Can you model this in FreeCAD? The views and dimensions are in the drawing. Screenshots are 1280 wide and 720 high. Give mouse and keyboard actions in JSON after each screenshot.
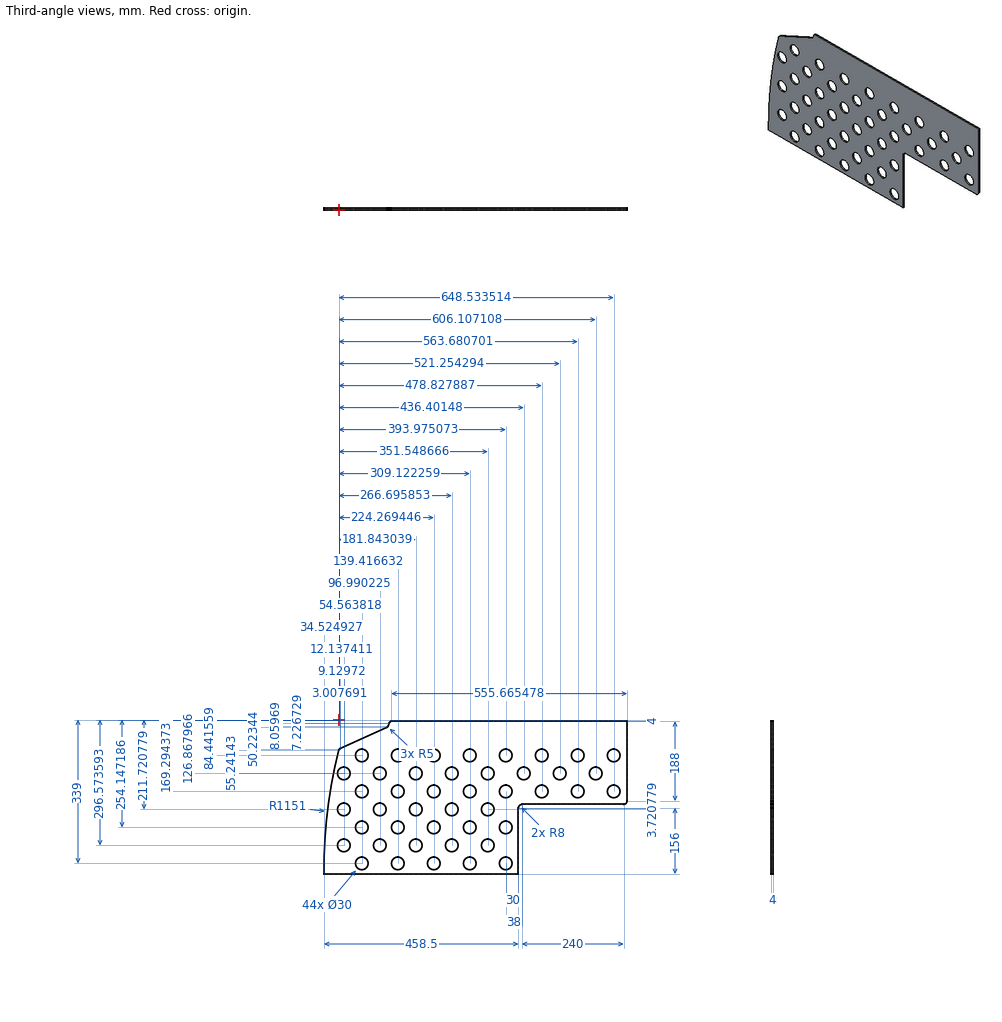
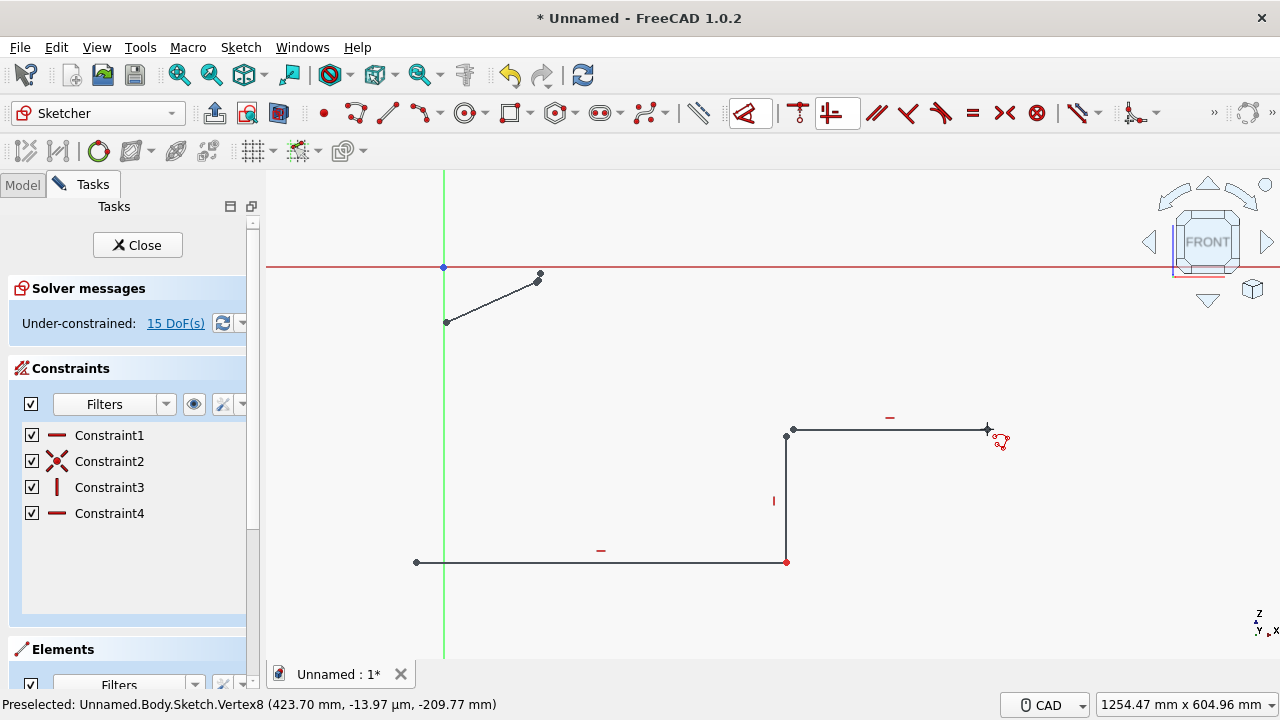
{"action": "scroll", "coordinate": [994, 423], "scroll_direction": "up", "scroll_amount": 3}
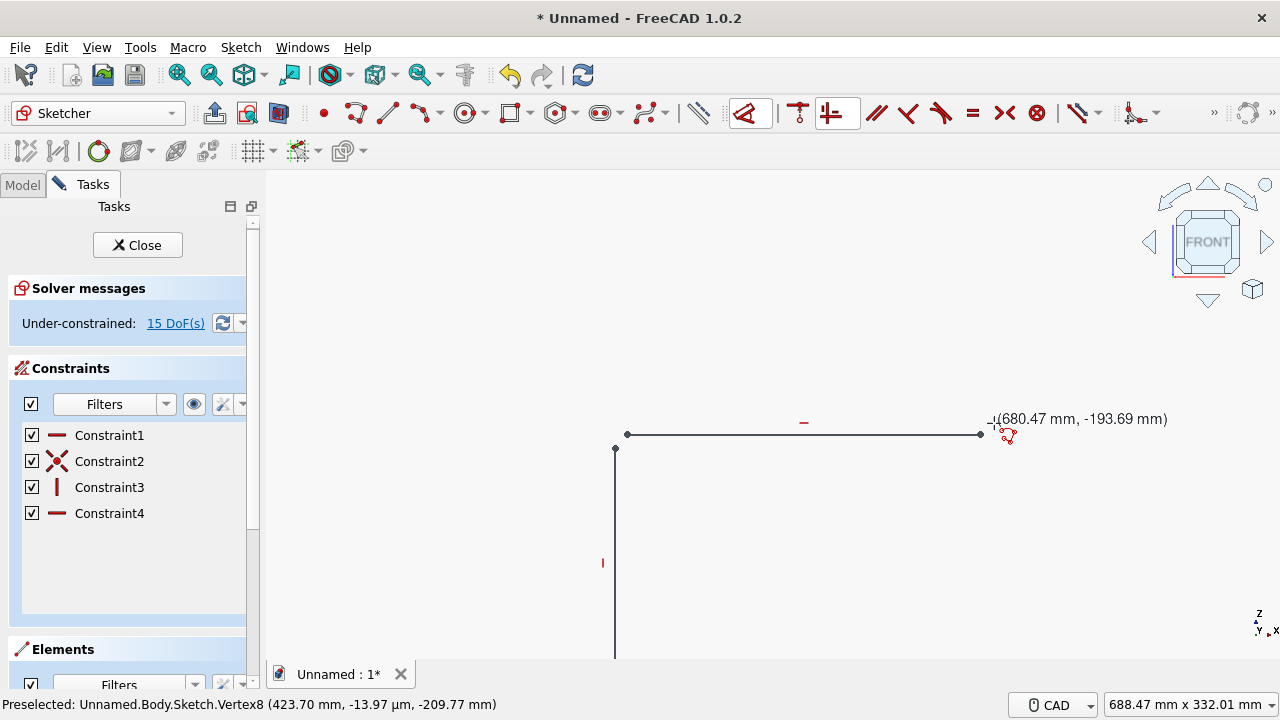
{"action": "left_click", "coordinate": [993, 422]}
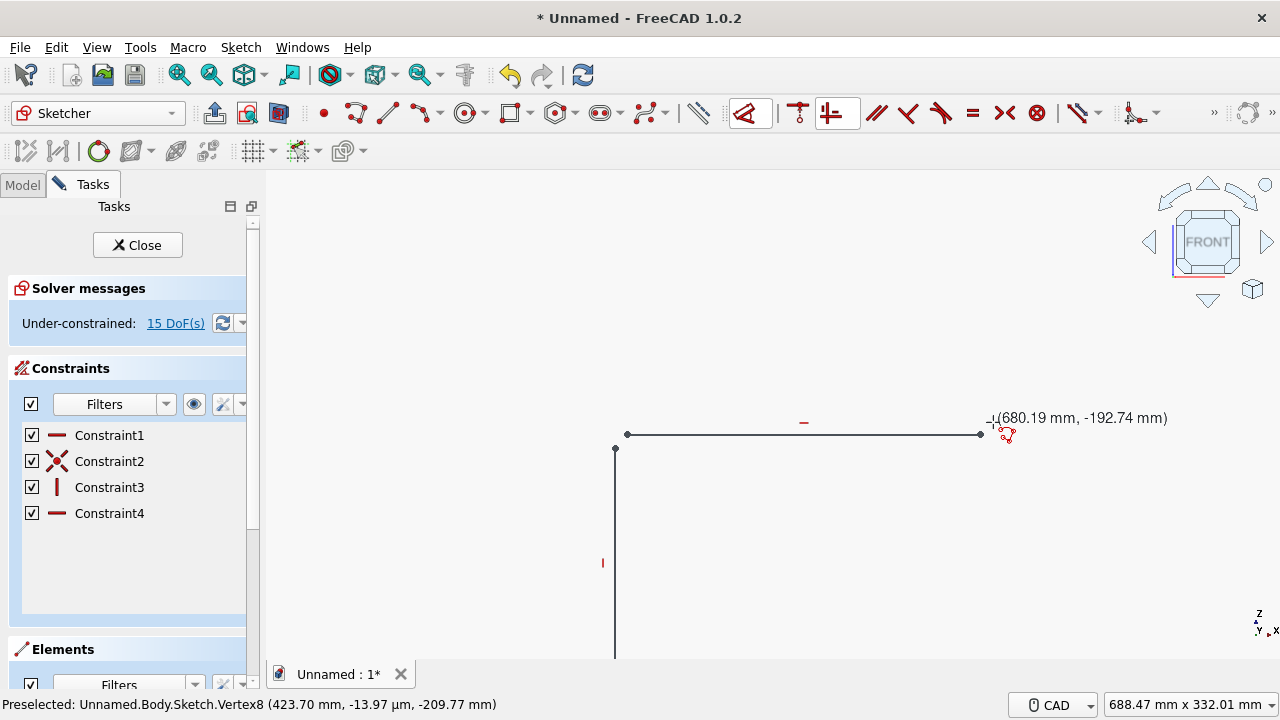
{"action": "scroll", "coordinate": [994, 423], "scroll_direction": "down", "scroll_amount": 3}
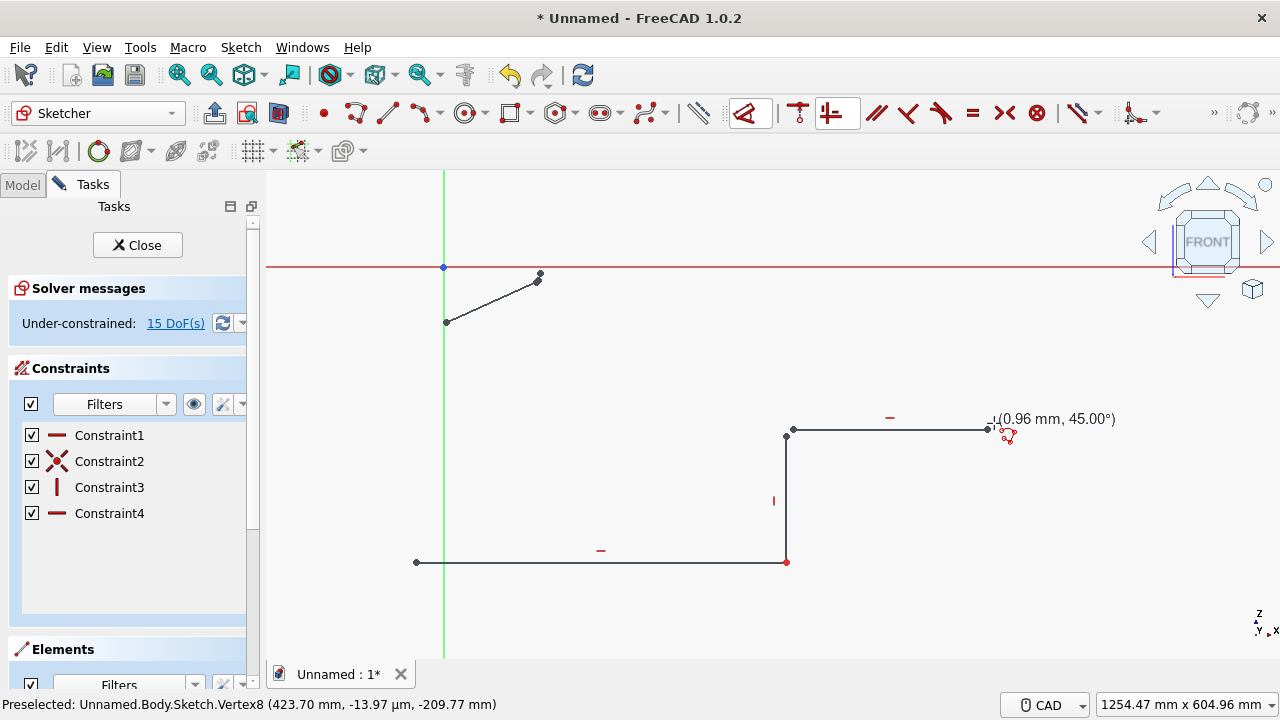
{"action": "scroll", "coordinate": [994, 271], "scroll_direction": "up", "scroll_amount": 8}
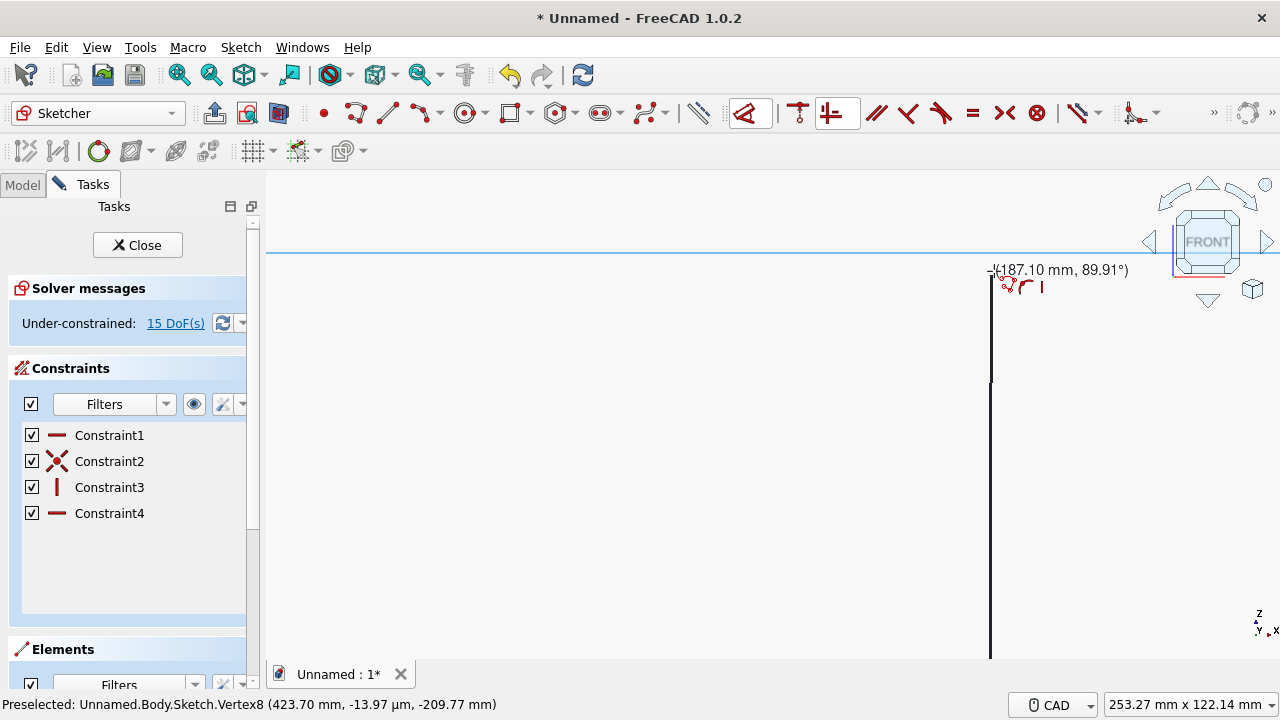
{"action": "left_click", "coordinate": [990, 269]}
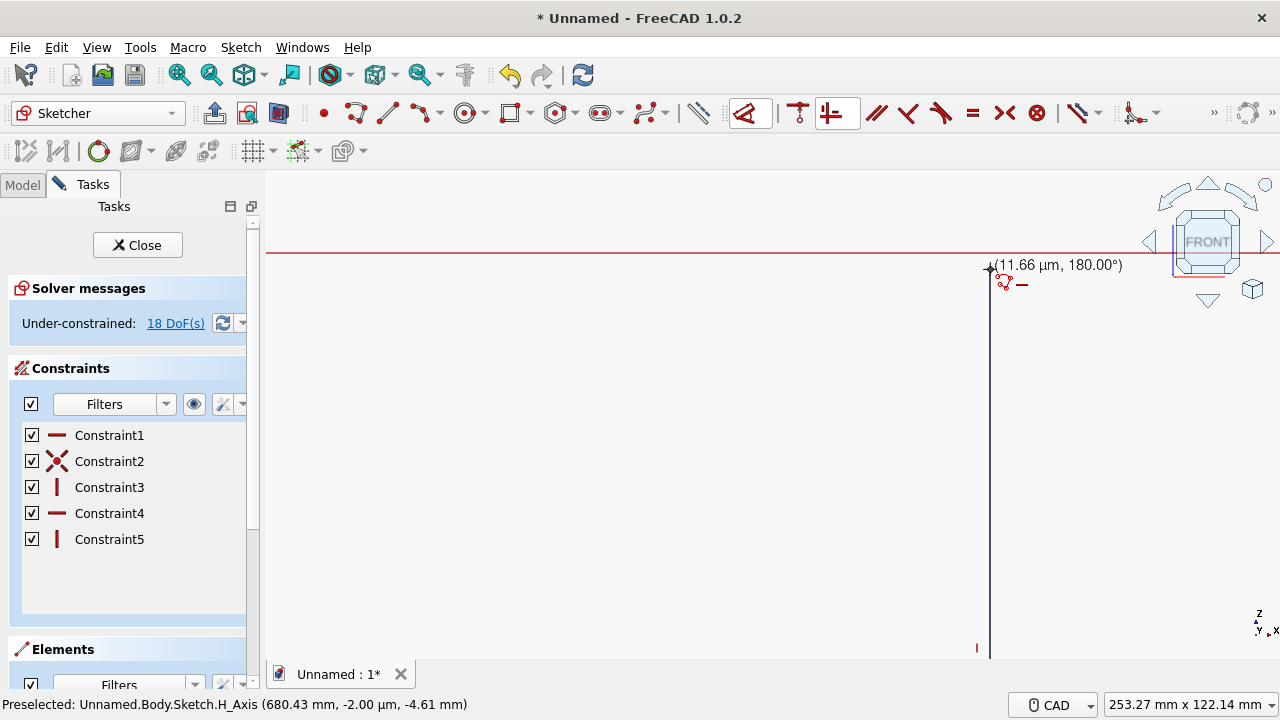
{"action": "scroll", "coordinate": [994, 271], "scroll_direction": "down", "scroll_amount": 8}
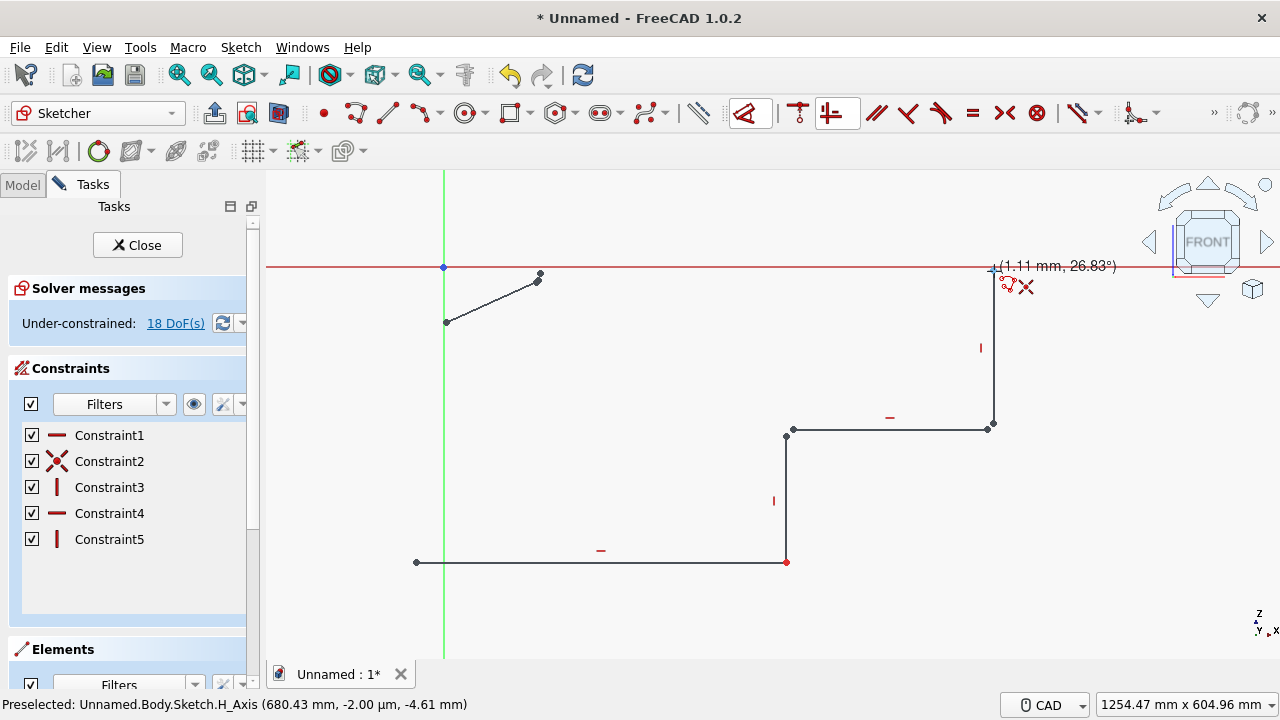
{"action": "scroll", "coordinate": [544, 271], "scroll_direction": "up", "scroll_amount": 8}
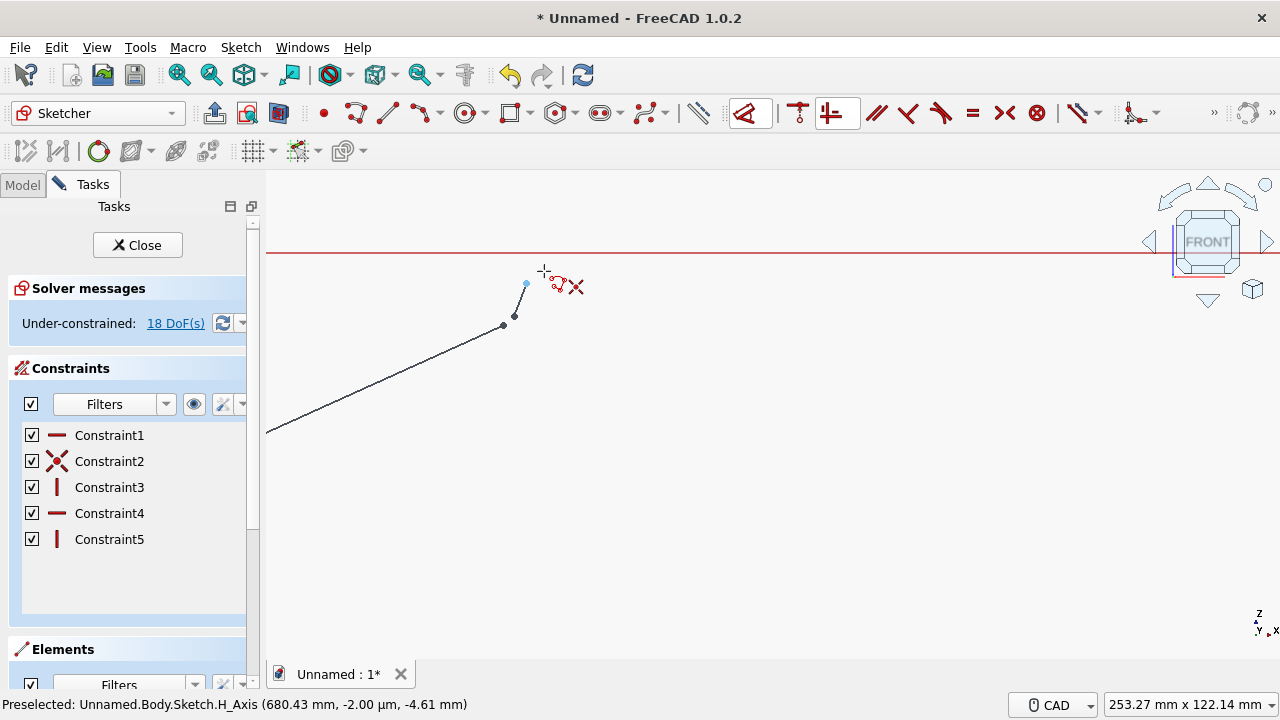
{"action": "left_click", "coordinate": [545, 269]}
{"action": "right_click", "coordinate": [545, 269]}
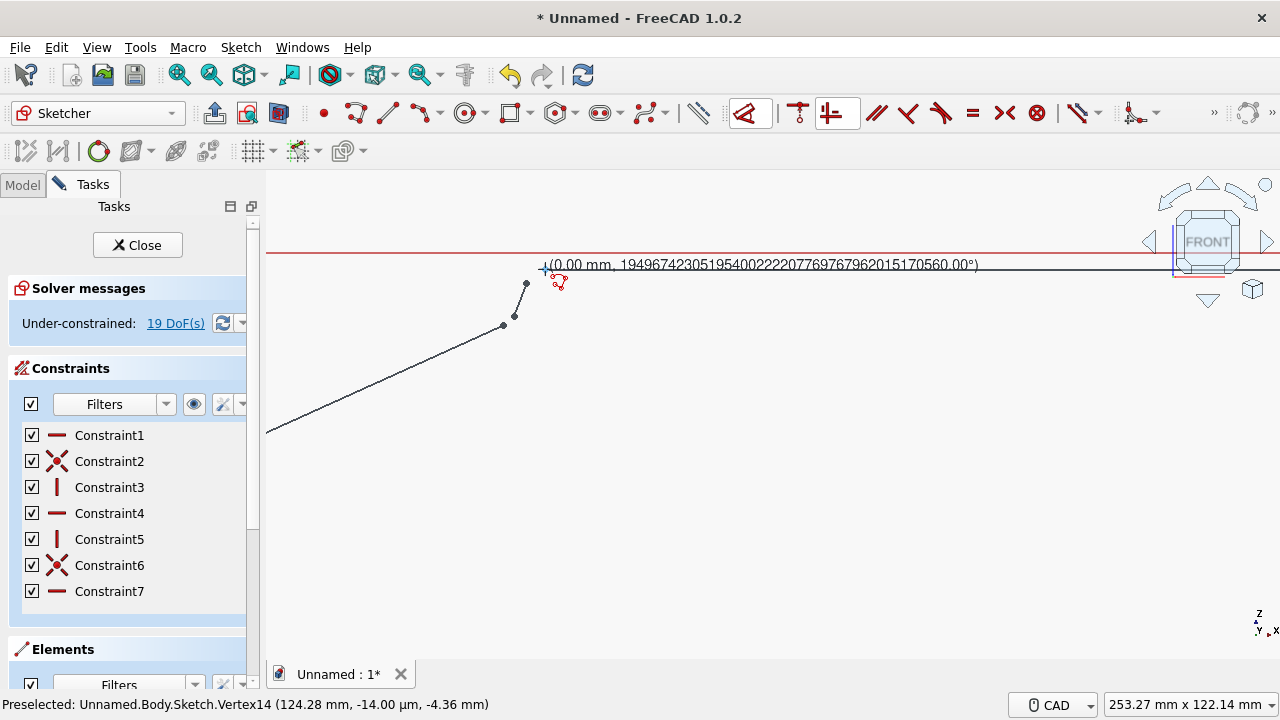
{"action": "key", "text": "g 3 a"}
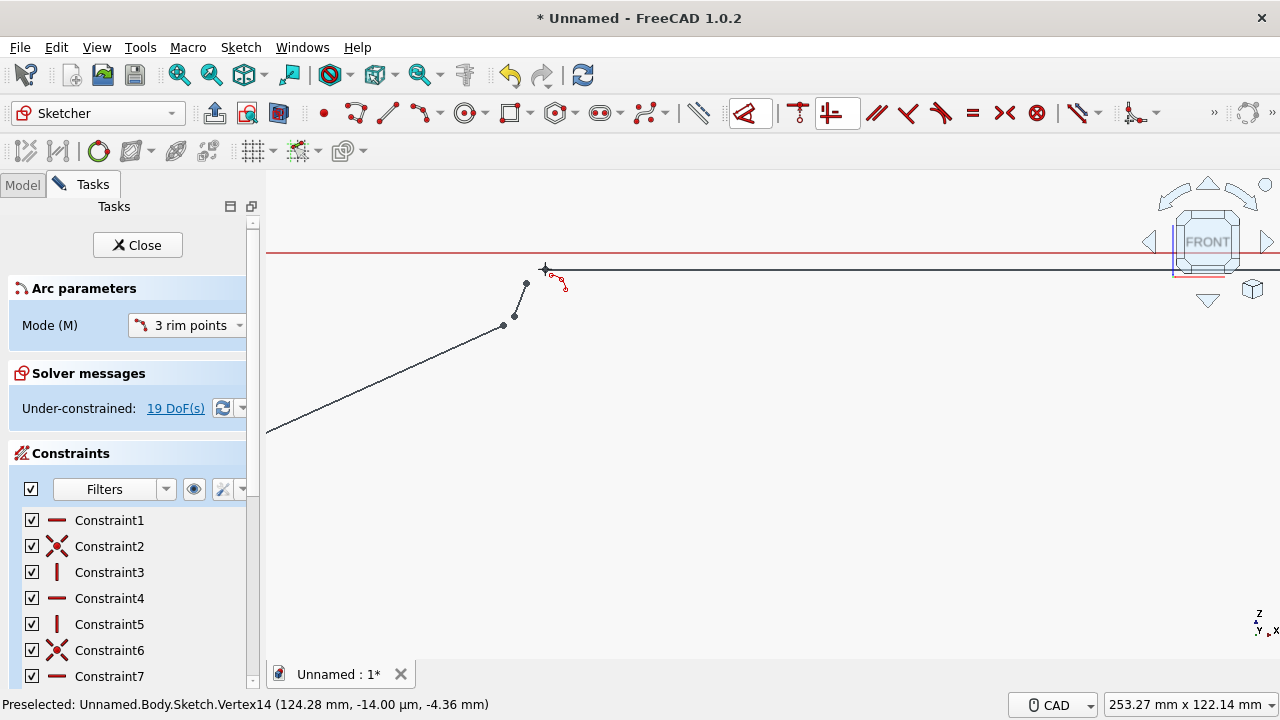
{"action": "left_click", "coordinate": [514, 316]}
{"action": "left_click", "coordinate": [503, 325]}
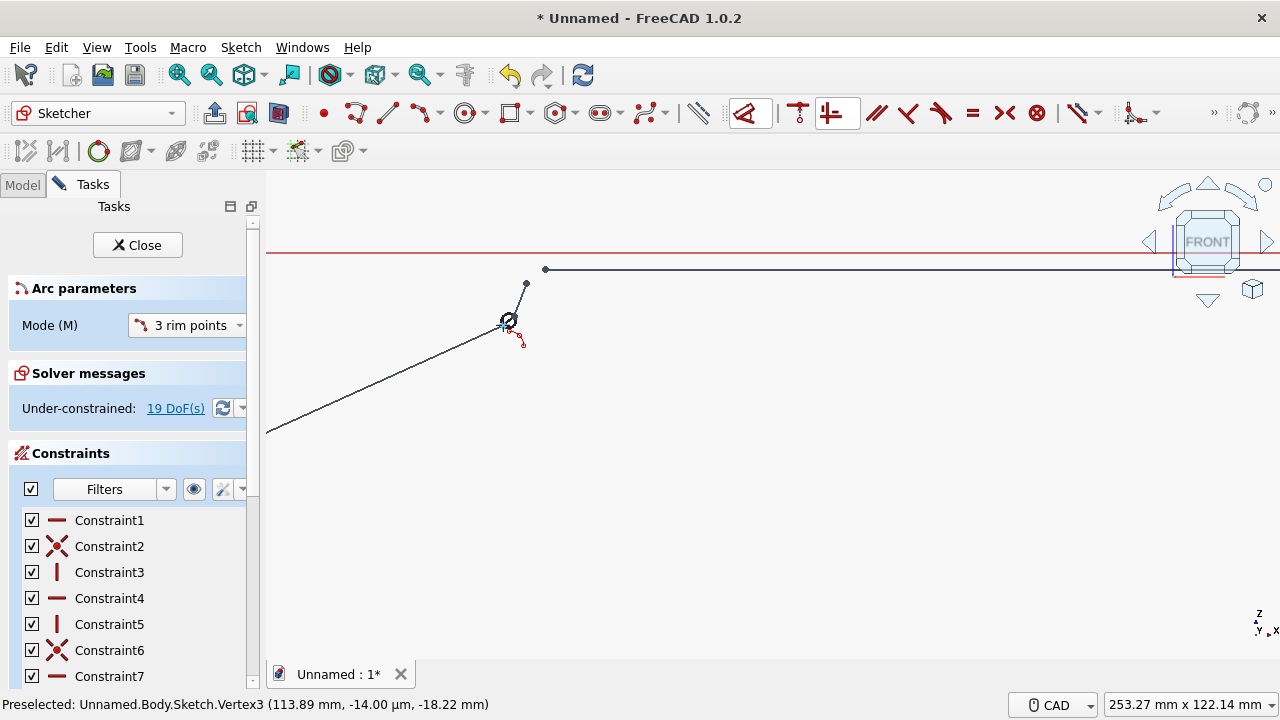
{"action": "scroll", "coordinate": [510, 320], "scroll_direction": "up", "scroll_amount": 12}